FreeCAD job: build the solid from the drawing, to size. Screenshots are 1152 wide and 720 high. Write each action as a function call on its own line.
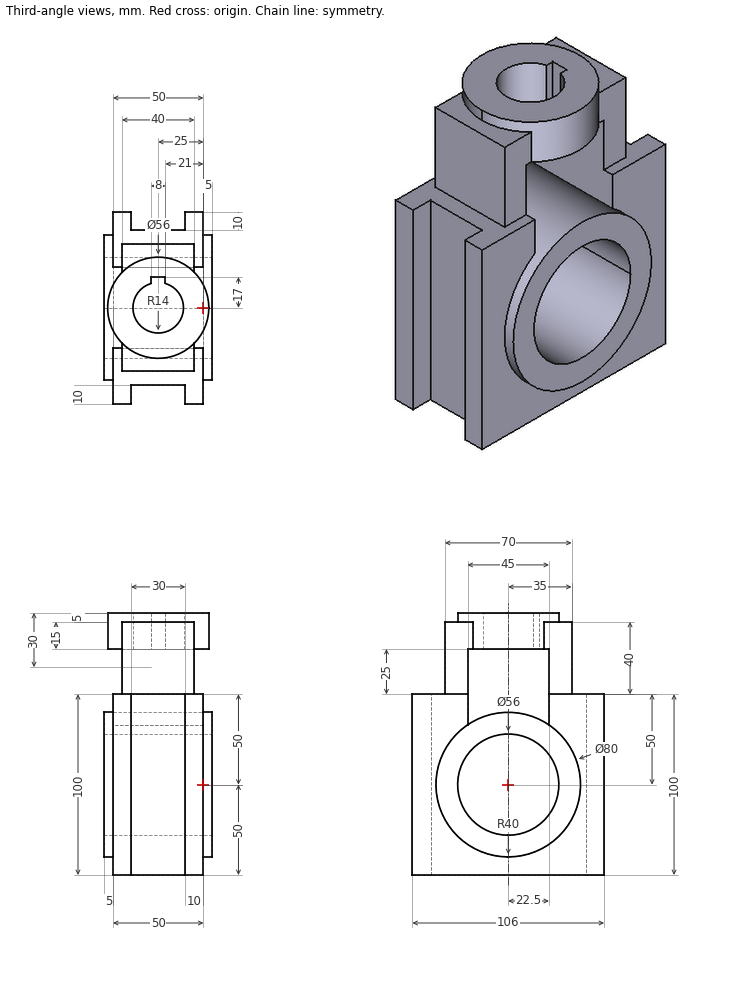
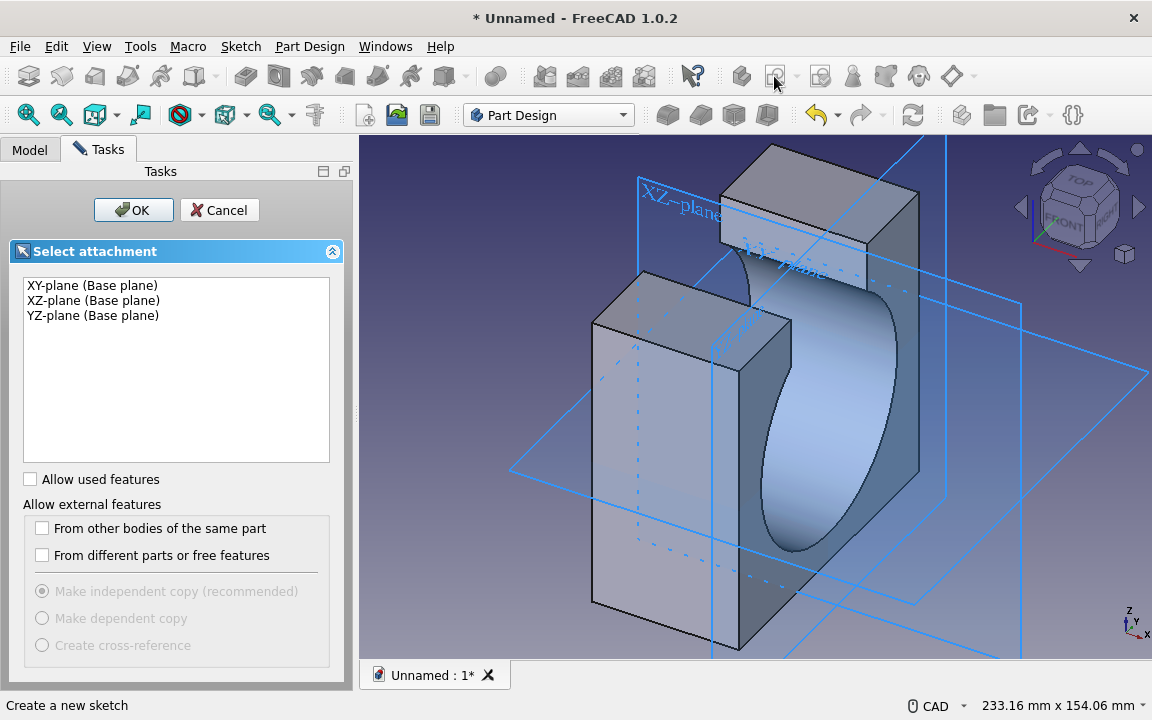
click(84, 316)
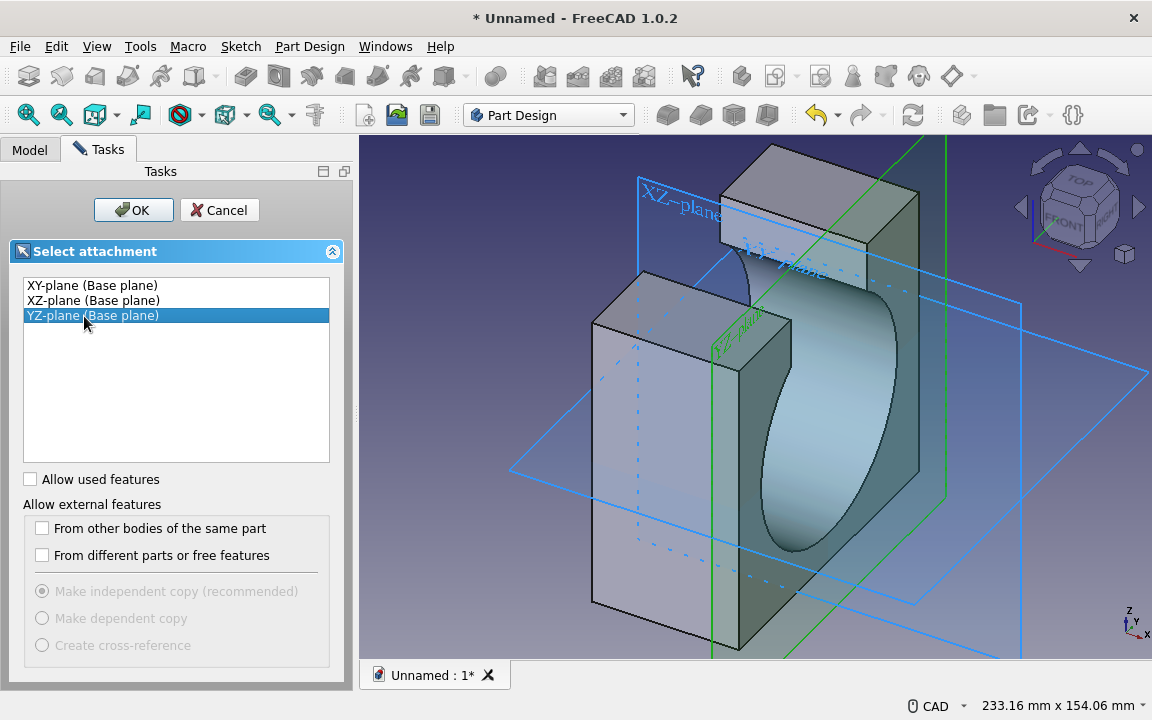
click(134, 210)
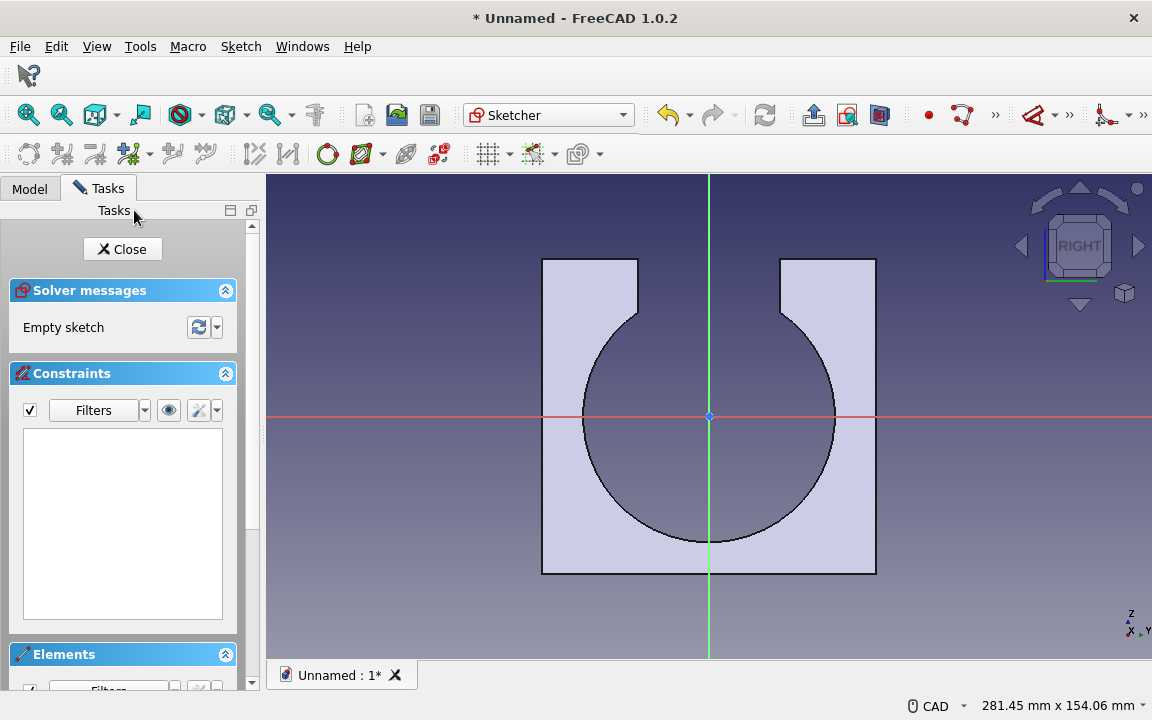
key(g)
key(c)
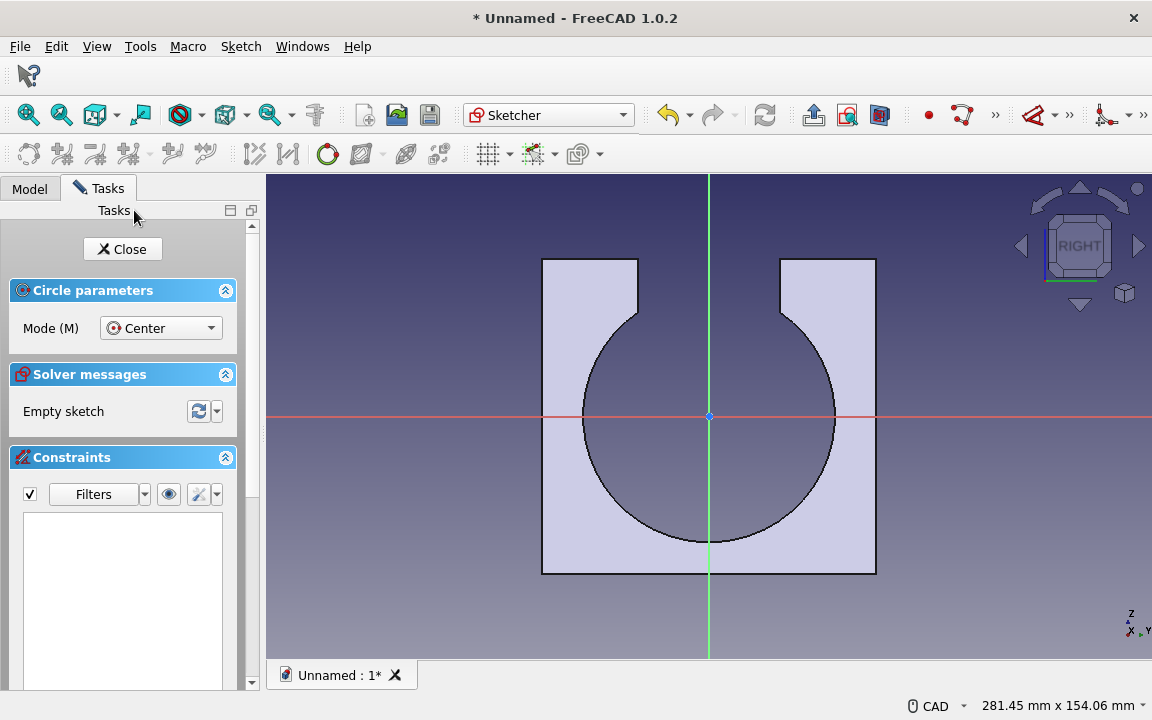
click(709, 416)
move(798, 327)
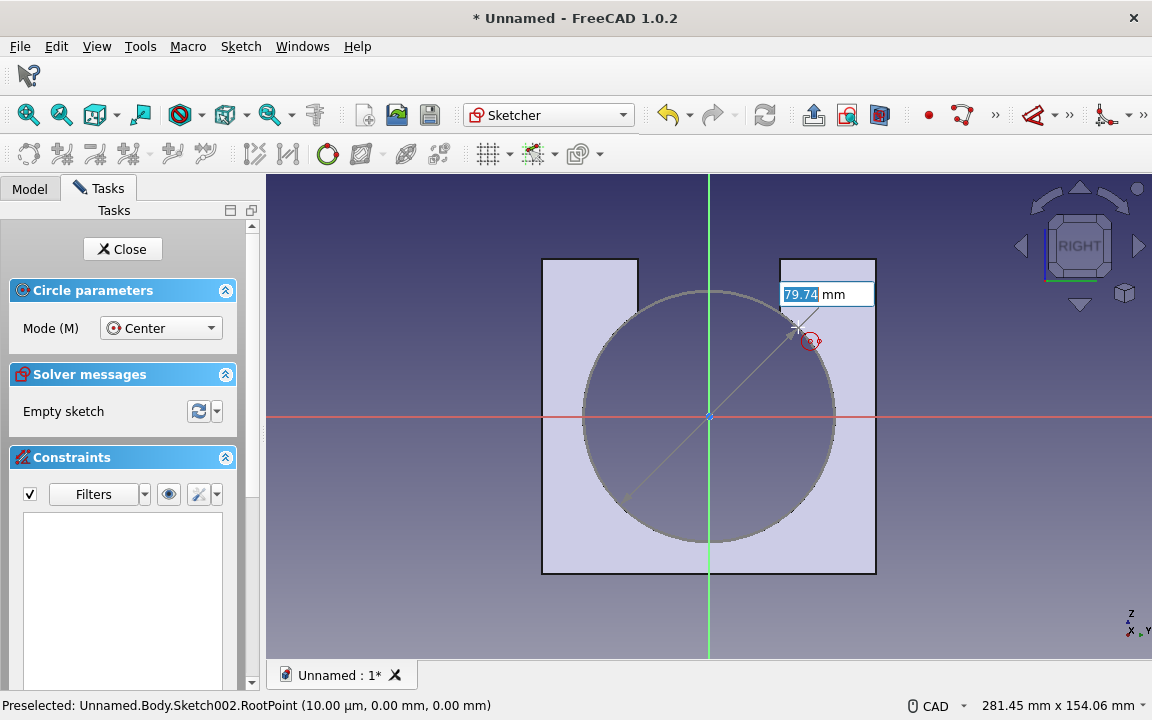
text(80)
key(Return)
key(Escape)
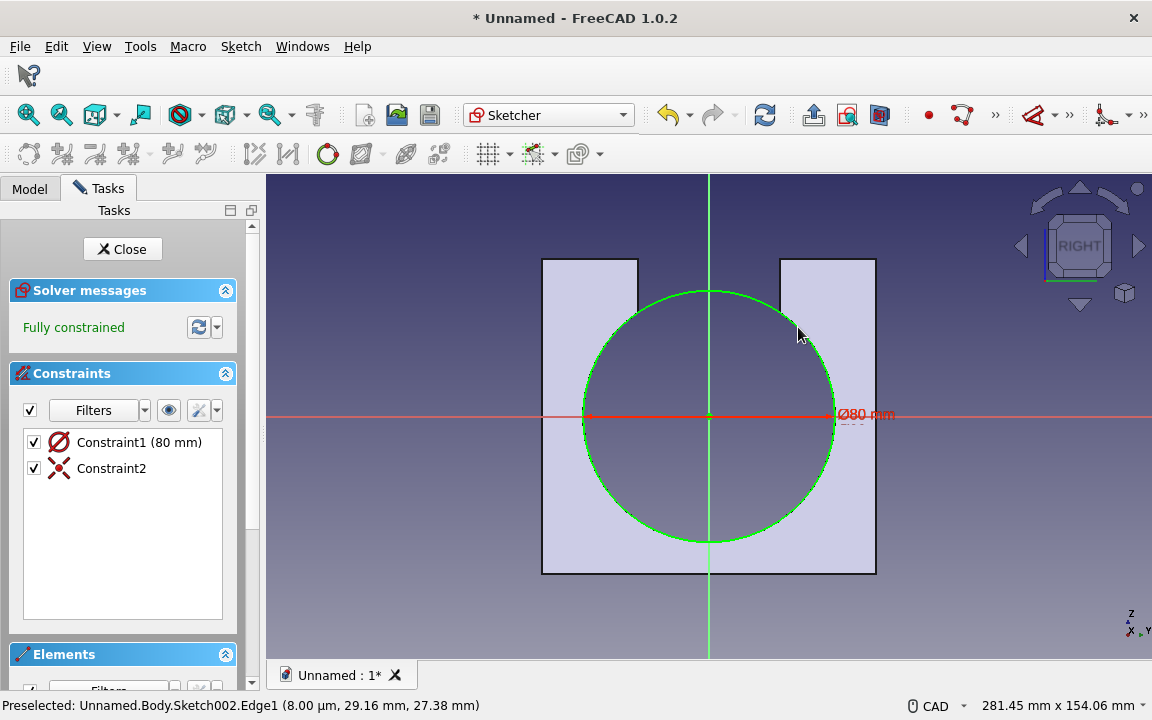
click(123, 249)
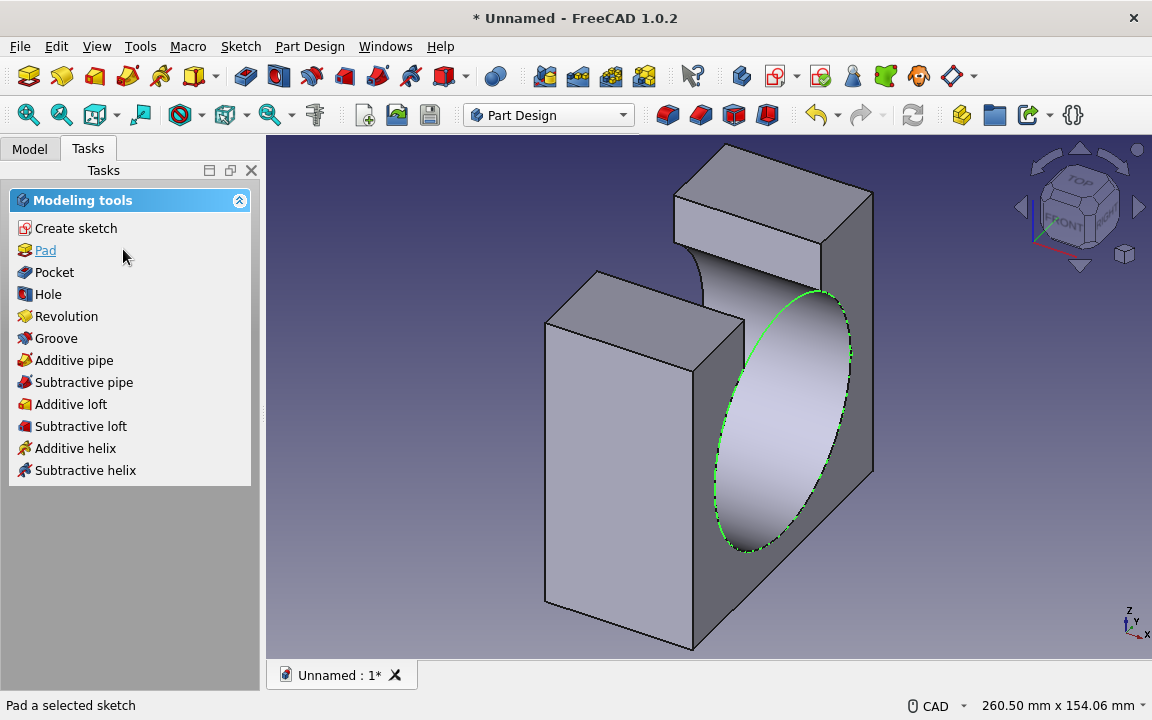
click(29, 76)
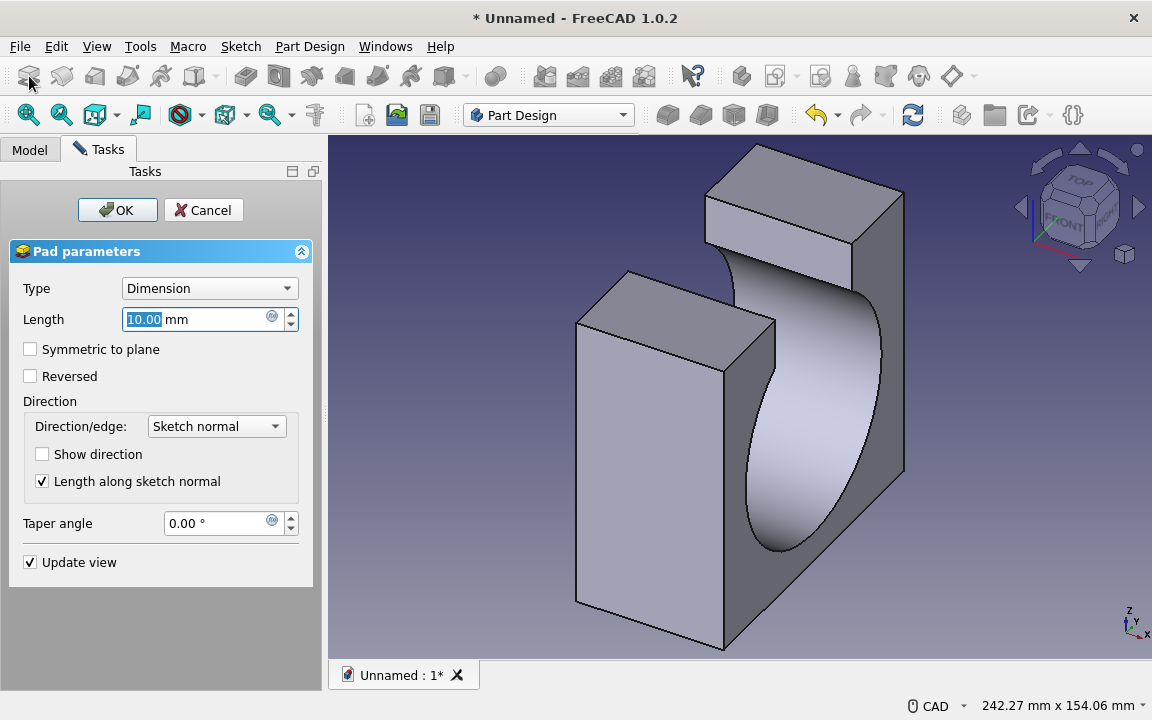
text(50)
key(Tab)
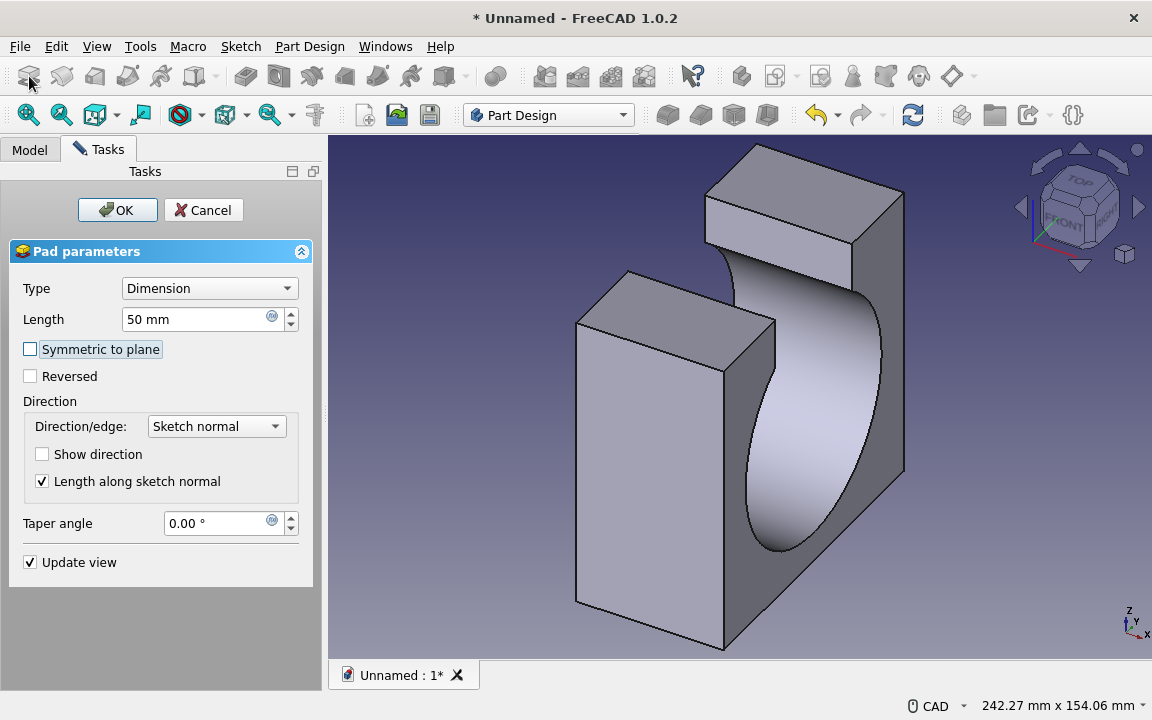
click(31, 376)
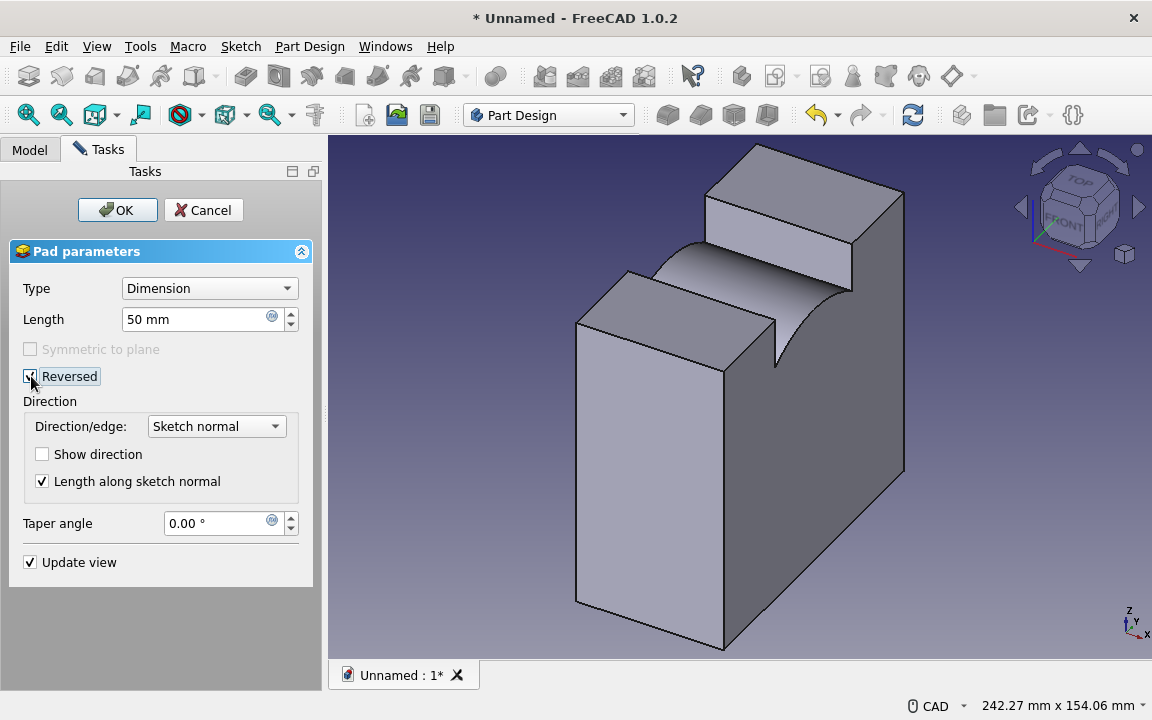
click(118, 210)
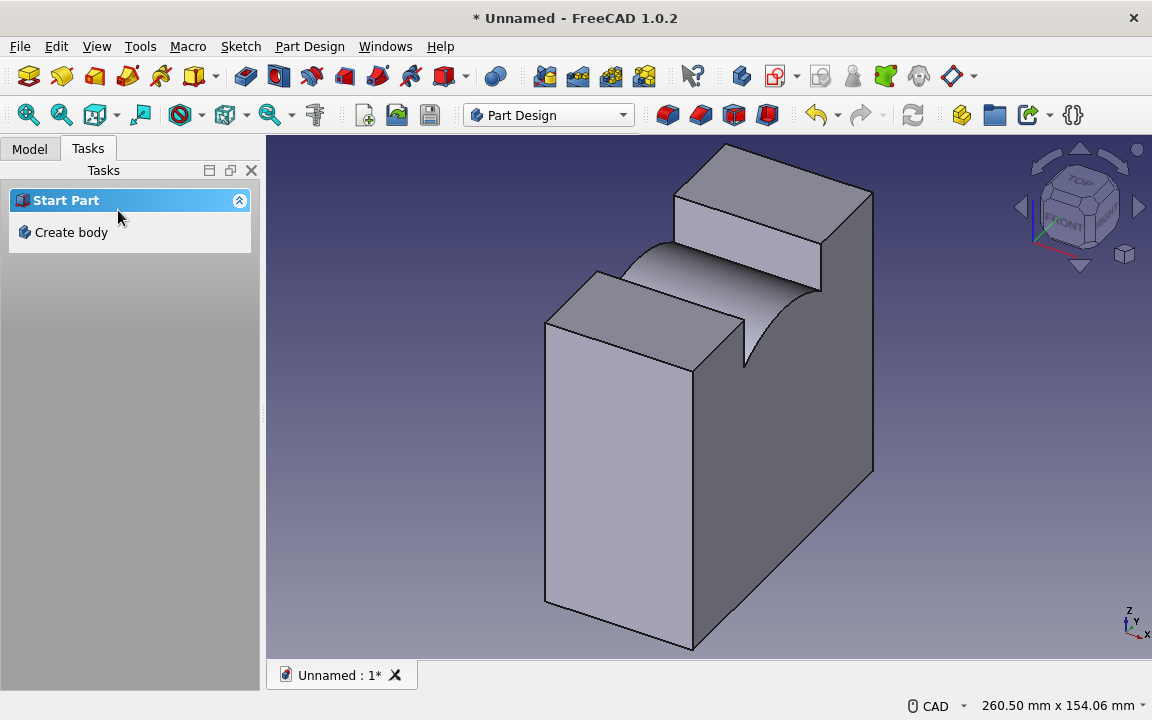
click(30, 148)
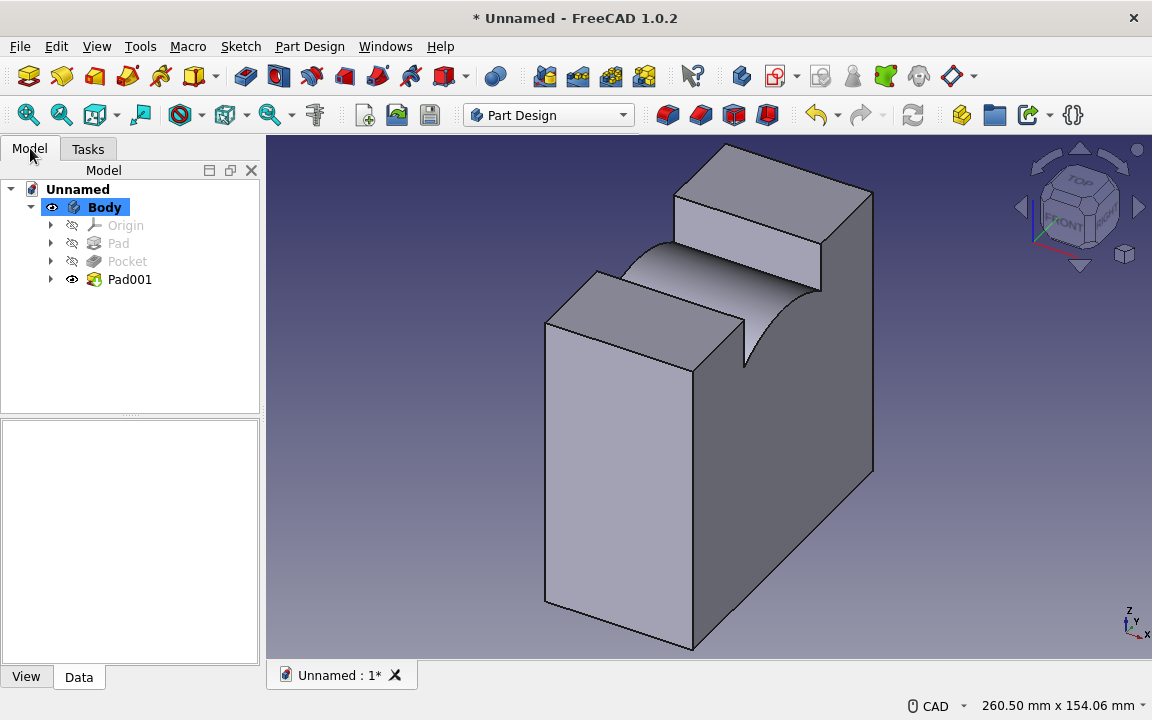
click(51, 225)